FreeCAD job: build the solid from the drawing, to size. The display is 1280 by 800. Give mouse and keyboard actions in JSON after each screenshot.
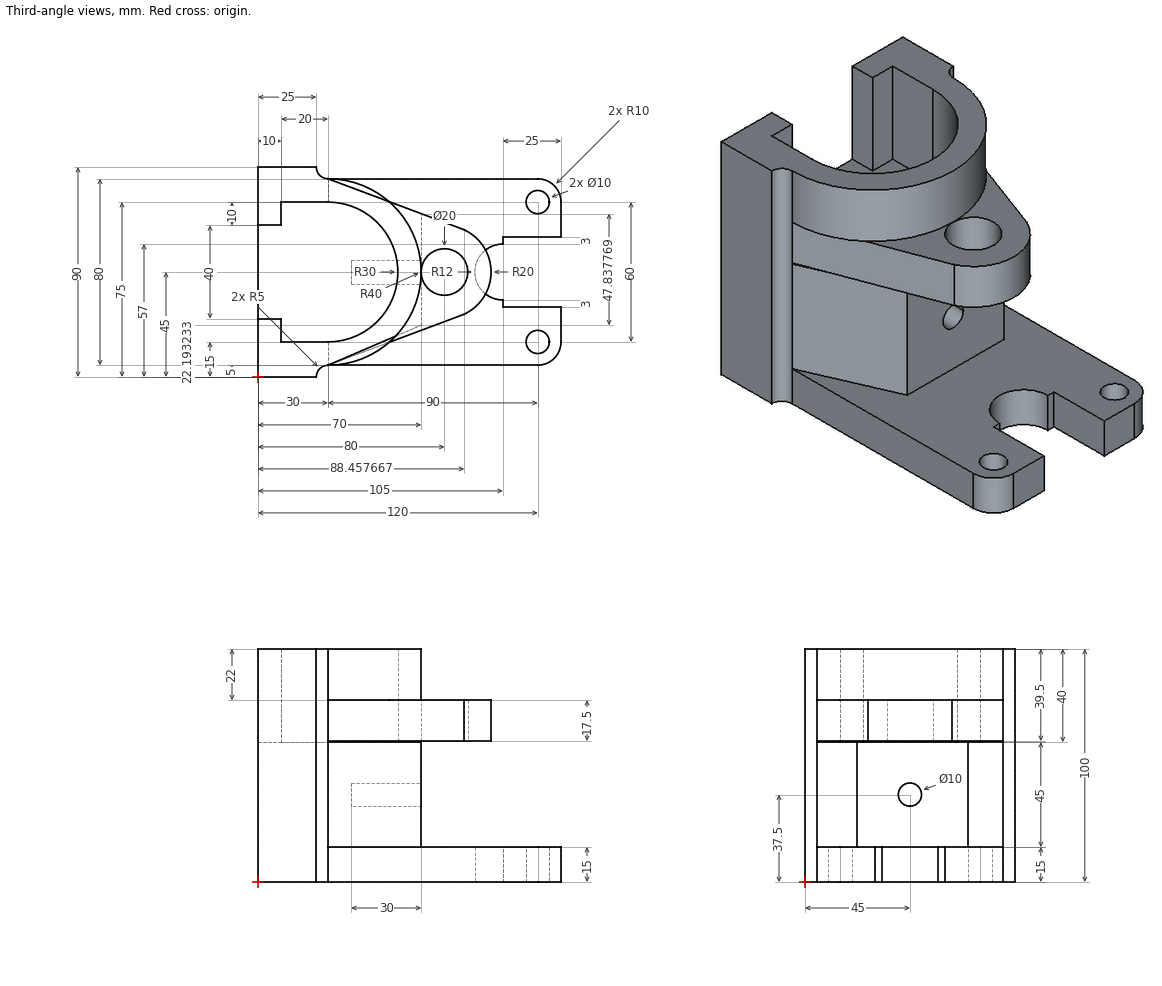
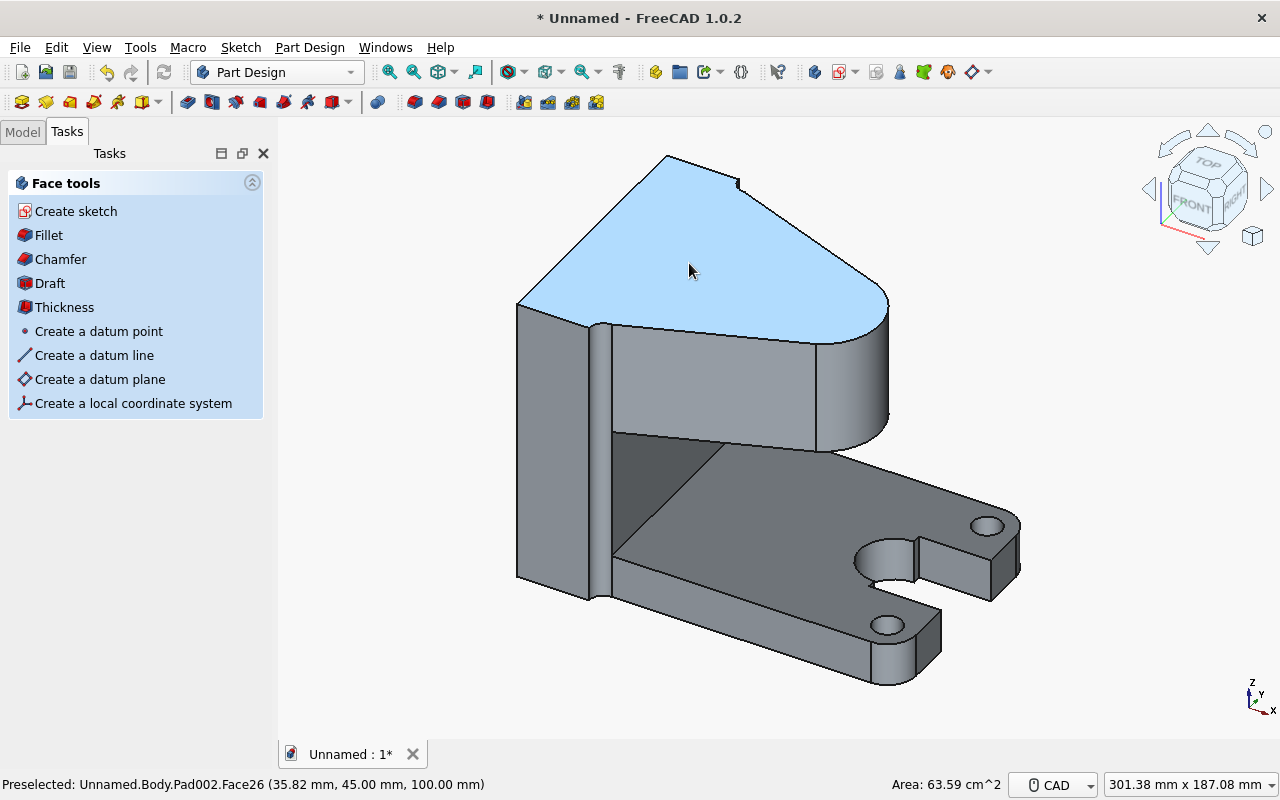
{"action": "left_click", "coordinate": [840, 72]}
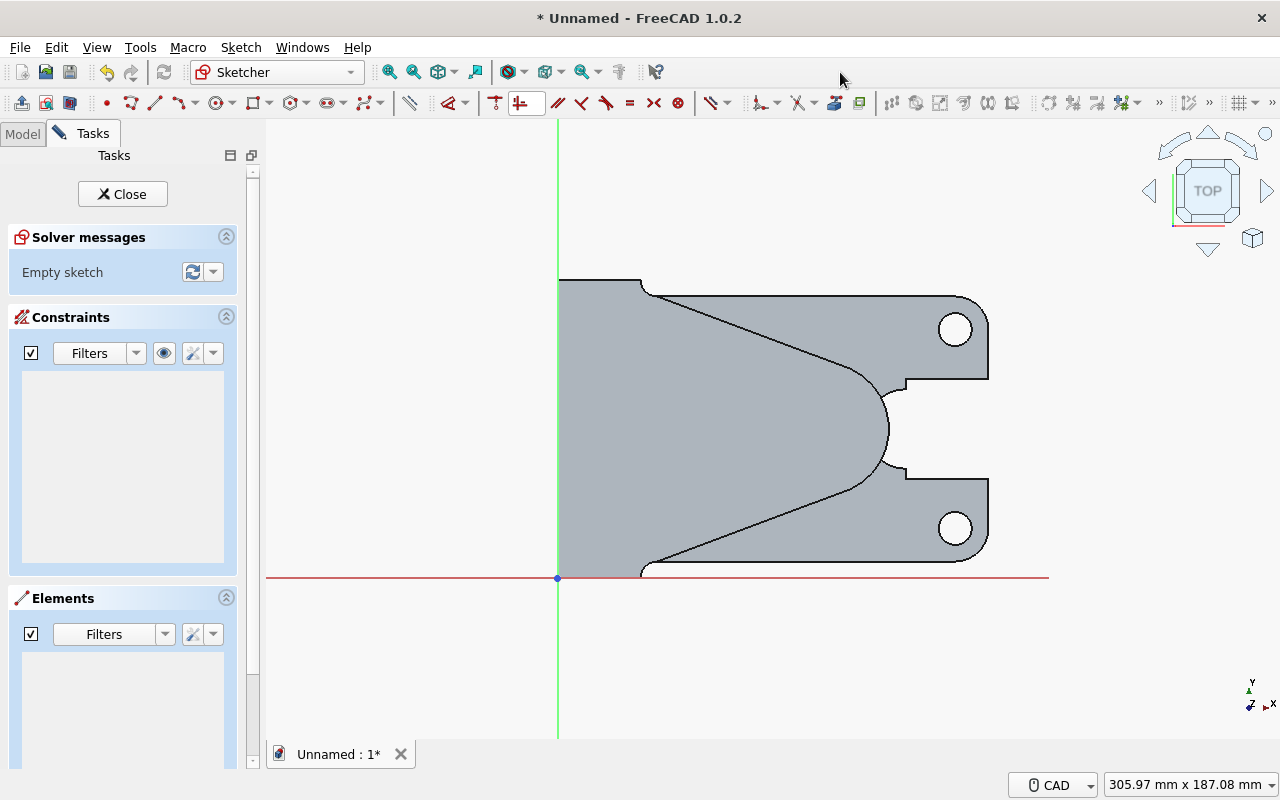
{"action": "scroll", "coordinate": [761, 454], "scroll_direction": "up", "scroll_amount": 2}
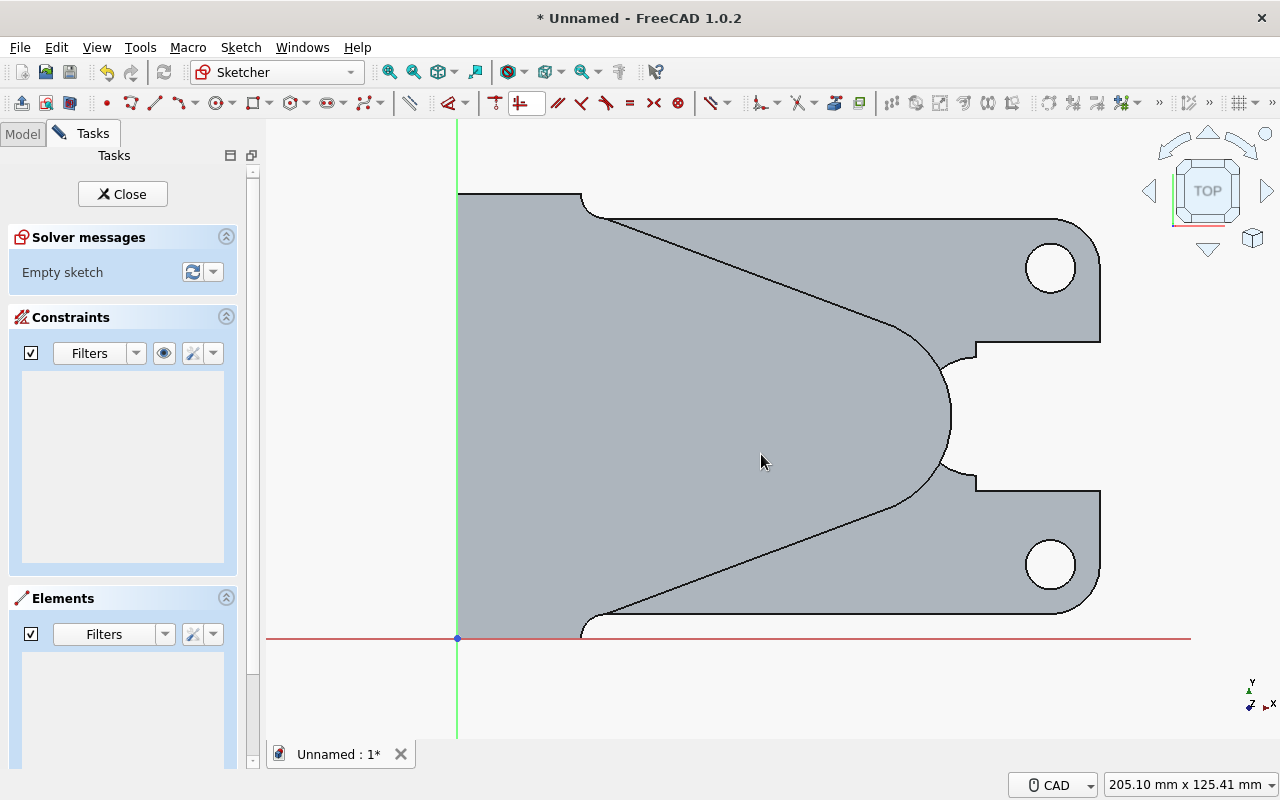
{"action": "key", "text": "g m"}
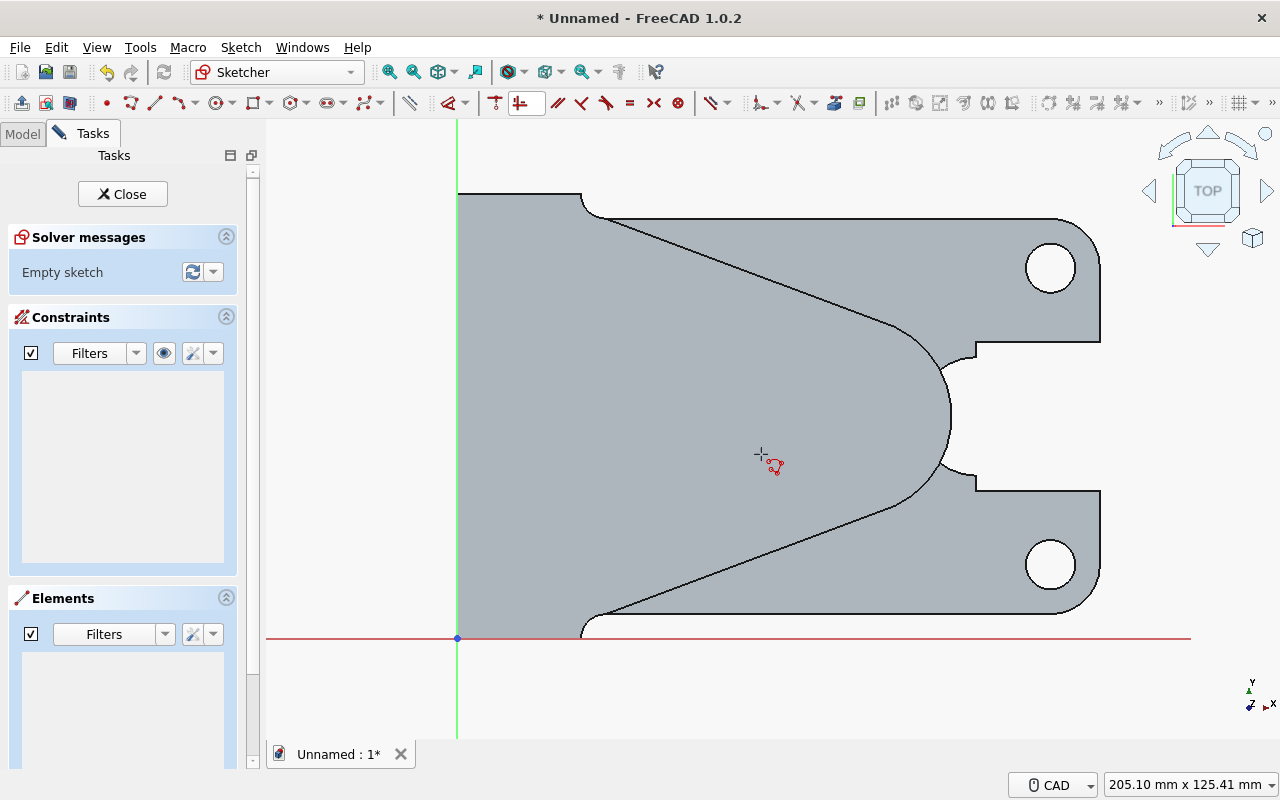
{"action": "left_click", "coordinate": [895, 327]}
{"action": "left_click", "coordinate": [606, 219]}
{"action": "left_click", "coordinate": [606, 614]}
{"action": "left_click", "coordinate": [895, 506]}
{"action": "right_click", "coordinate": [895, 506]}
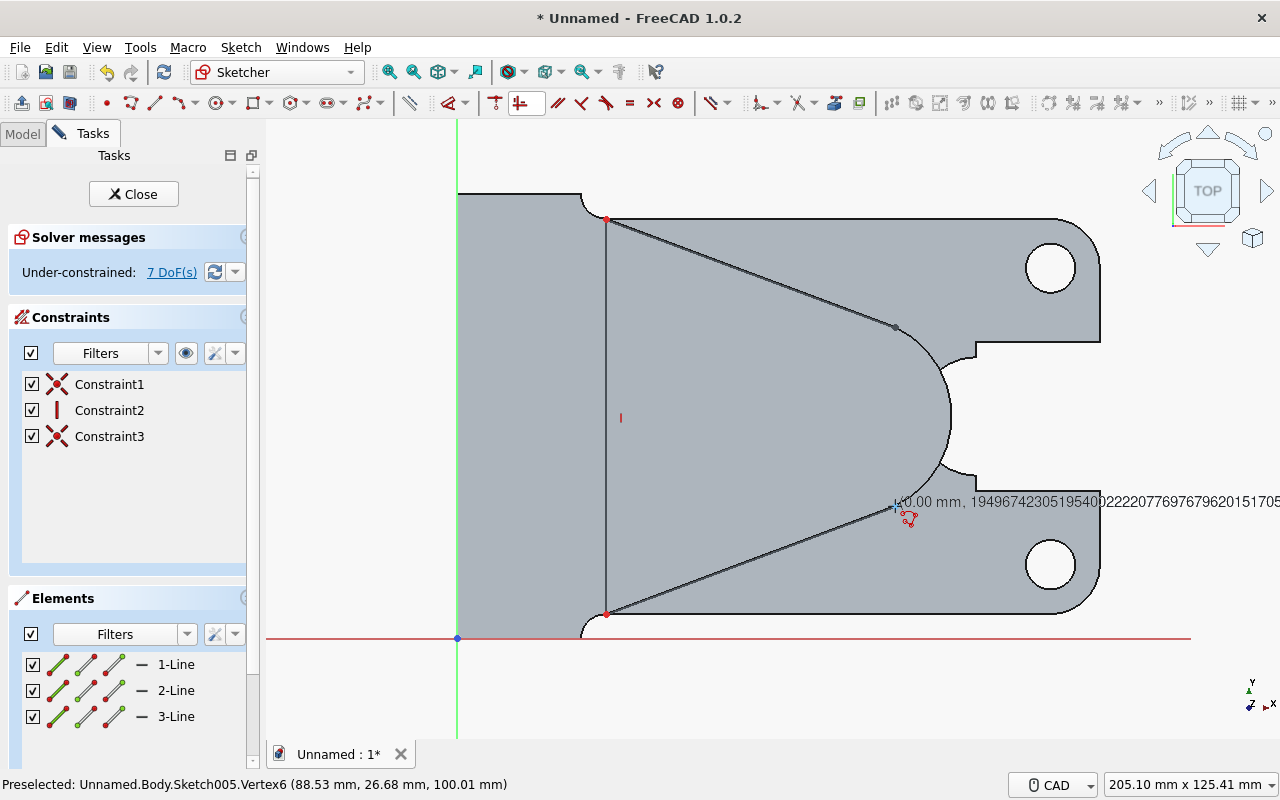
{"action": "key", "text": "g 3 a"}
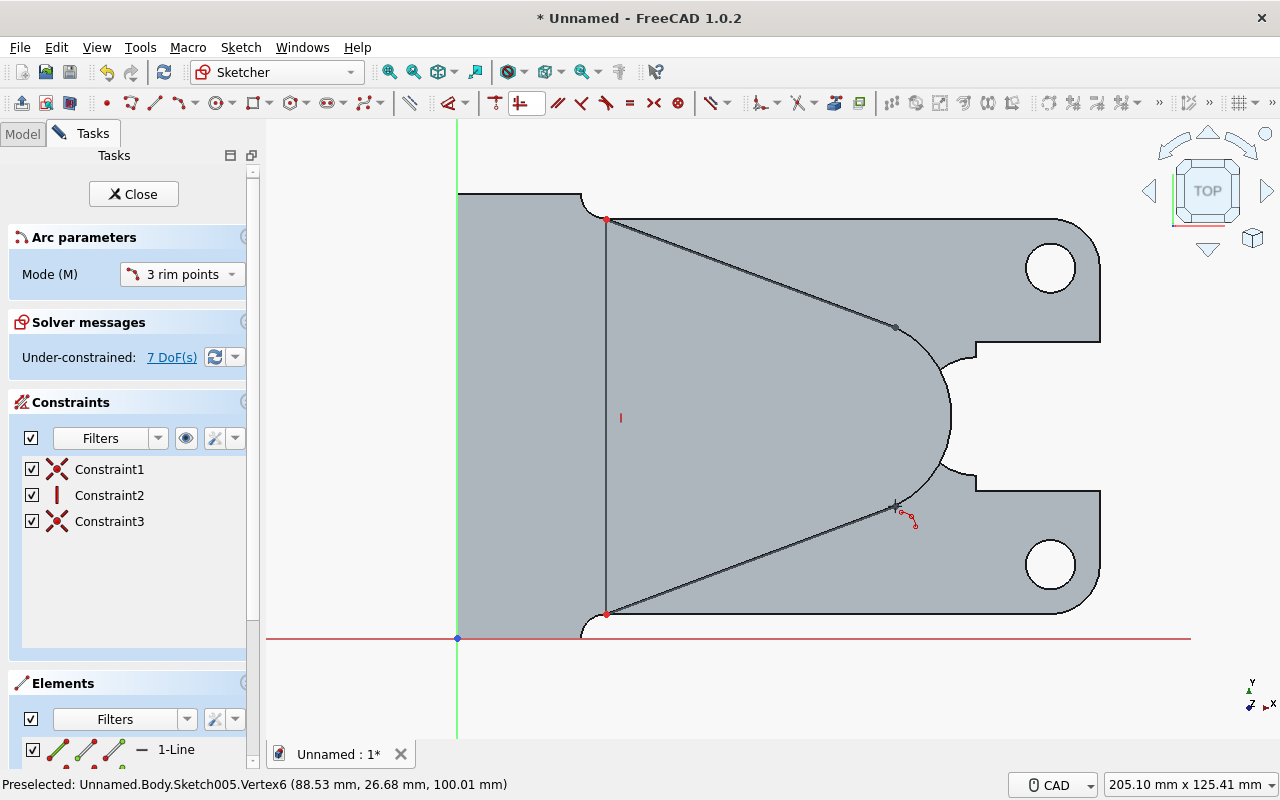
{"action": "left_click", "coordinate": [895, 507]}
{"action": "left_click", "coordinate": [895, 328]}
{"action": "left_click", "coordinate": [952, 416]}
{"action": "key", "text": "Escape"}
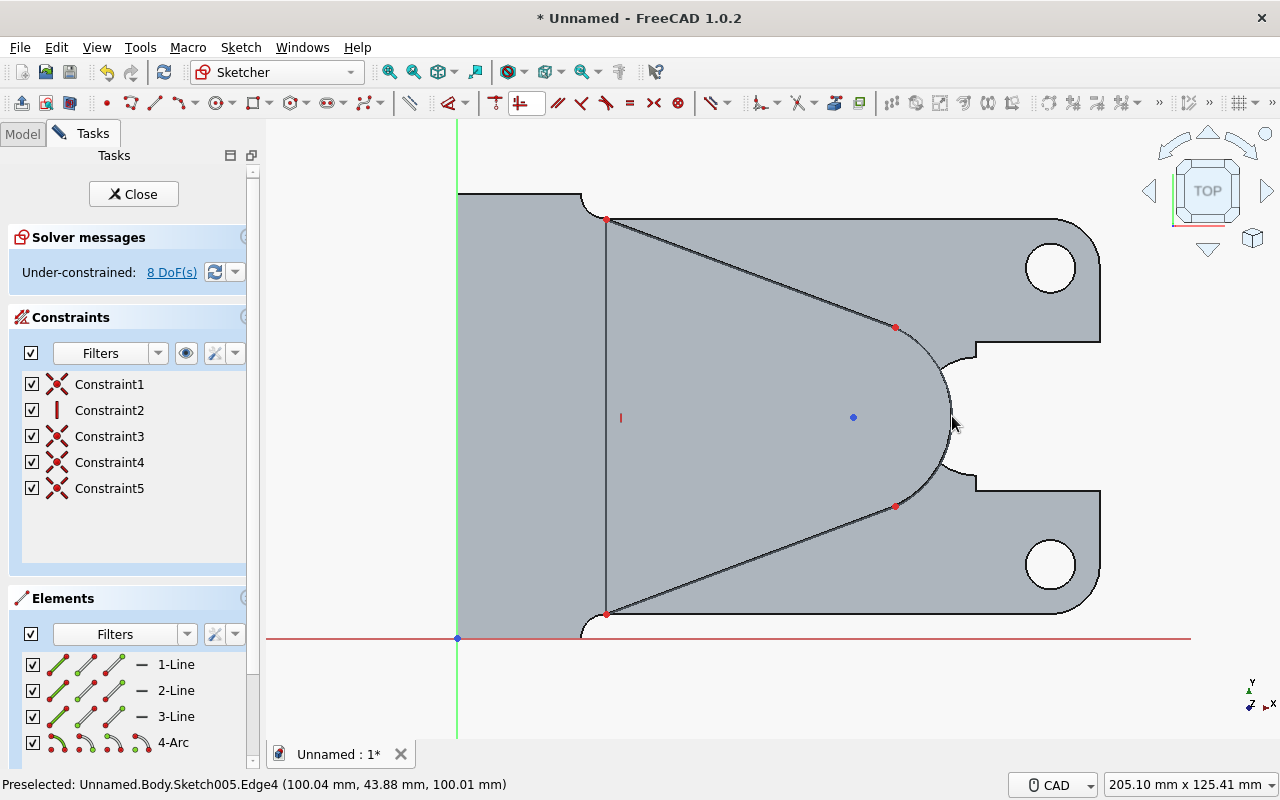
{"action": "left_click", "coordinate": [448, 104]}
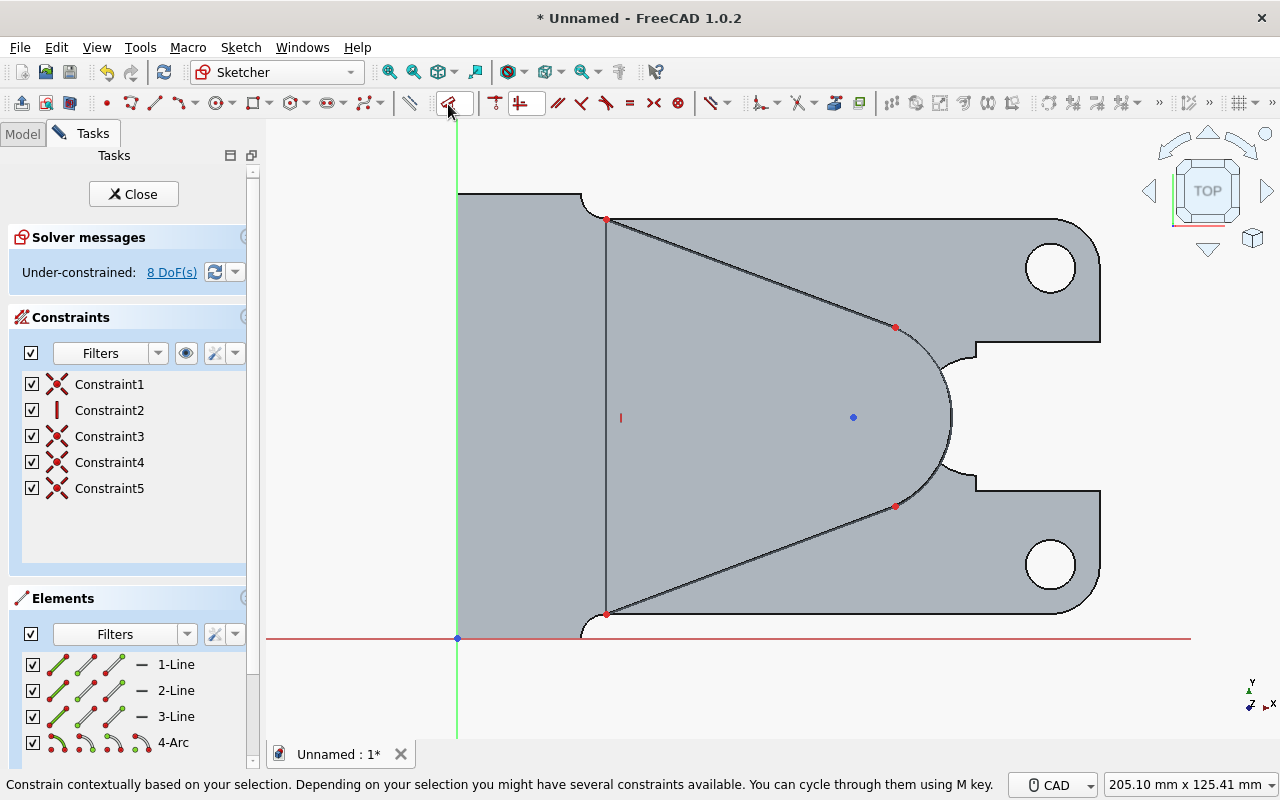
{"action": "left_click", "coordinate": [942, 461]}
{"action": "left_click", "coordinate": [971, 475]}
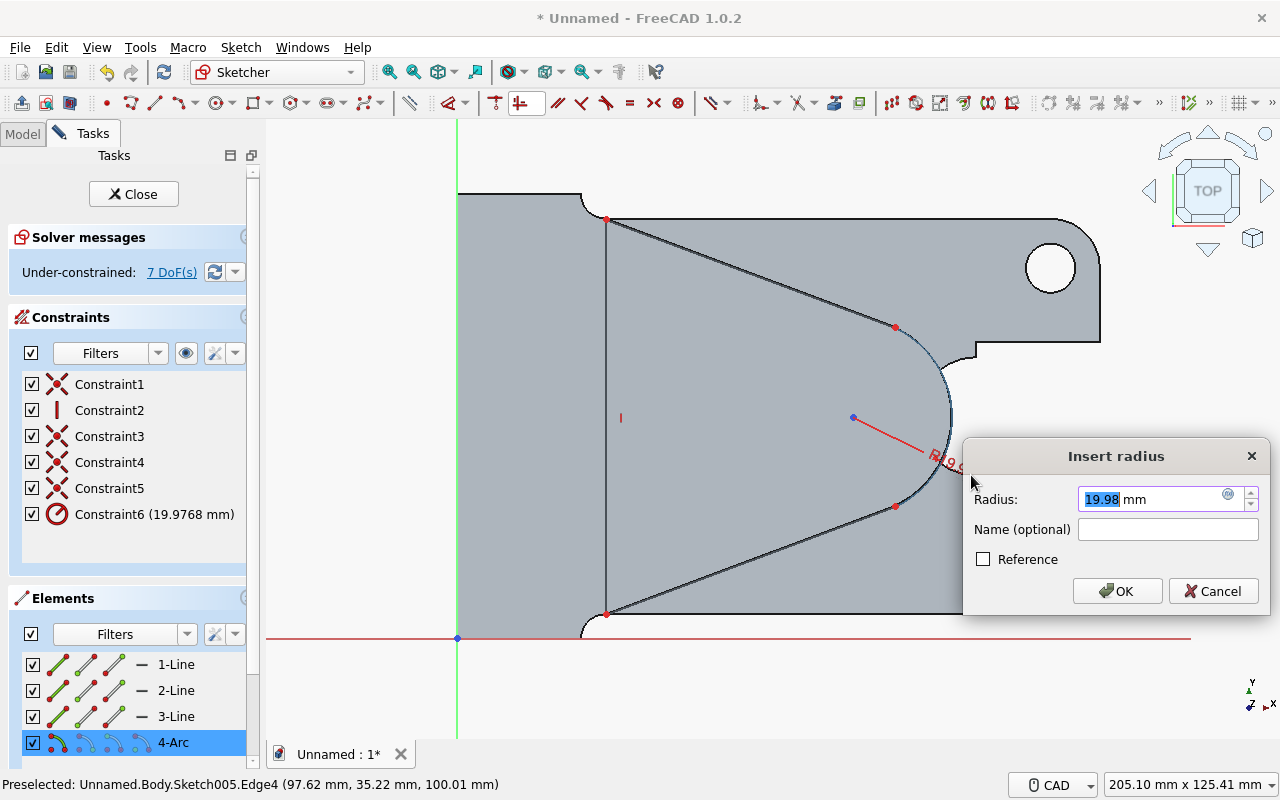
{"action": "type", "text": "20"}
{"action": "key", "text": "Return"}